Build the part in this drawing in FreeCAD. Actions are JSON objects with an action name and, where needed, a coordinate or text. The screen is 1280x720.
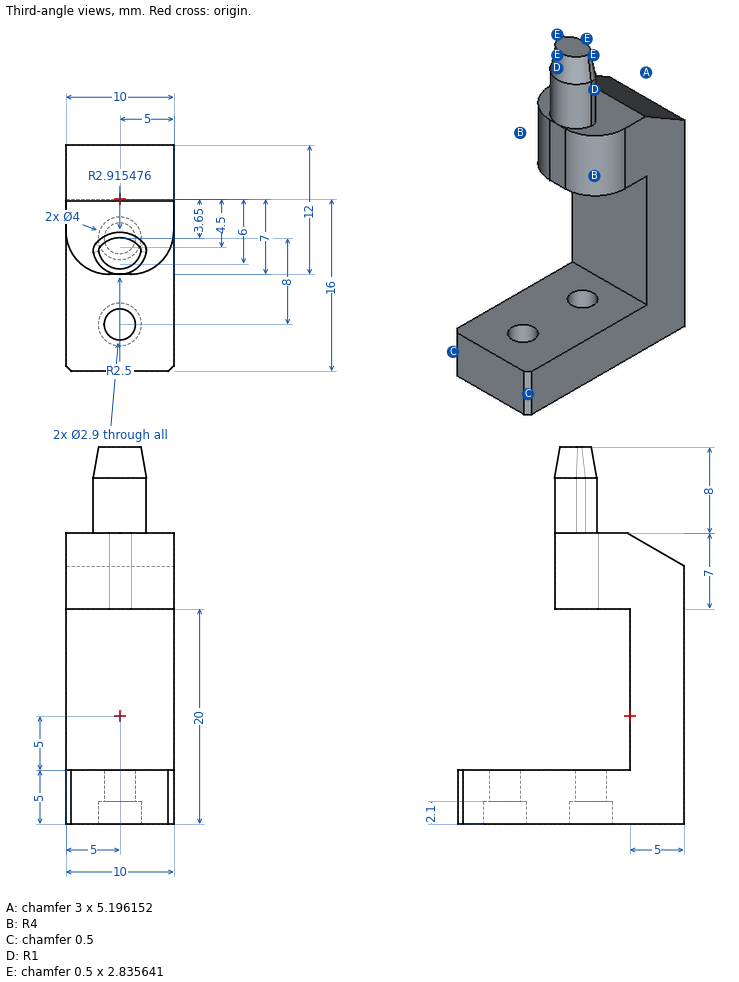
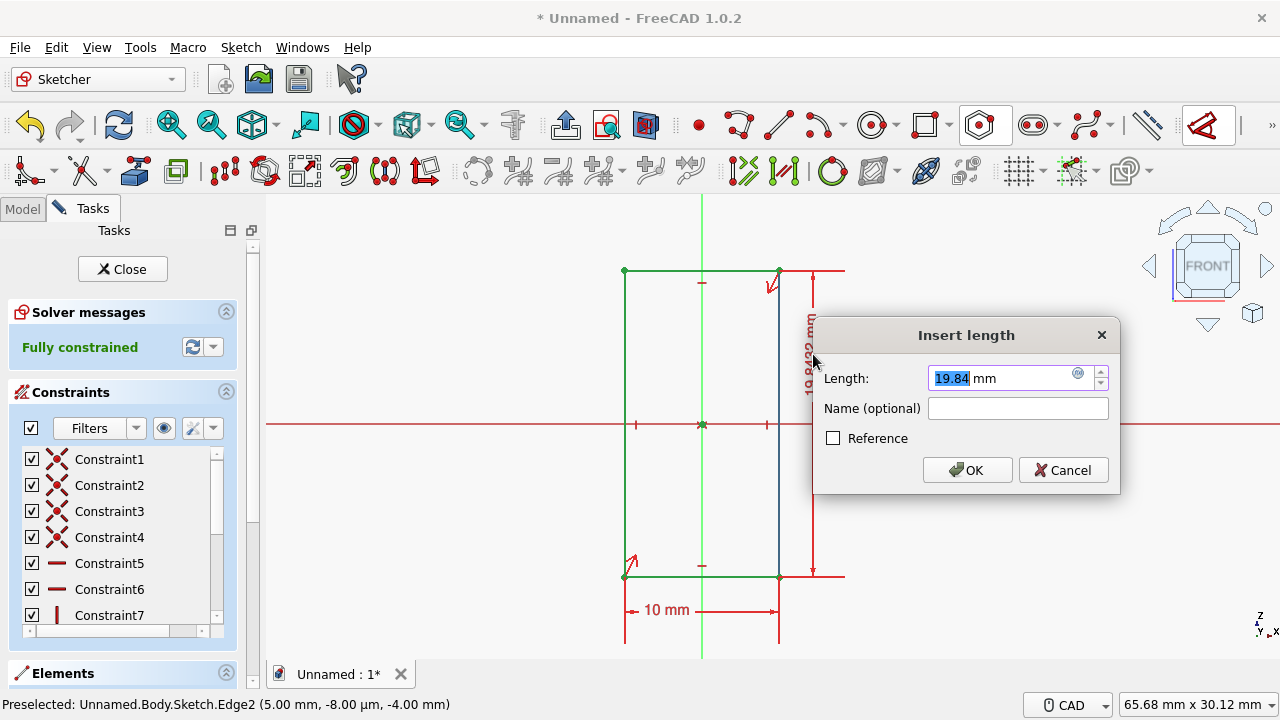
{"action": "type", "text": "20"}
{"action": "key", "text": "Return"}
{"action": "key", "text": "Escape"}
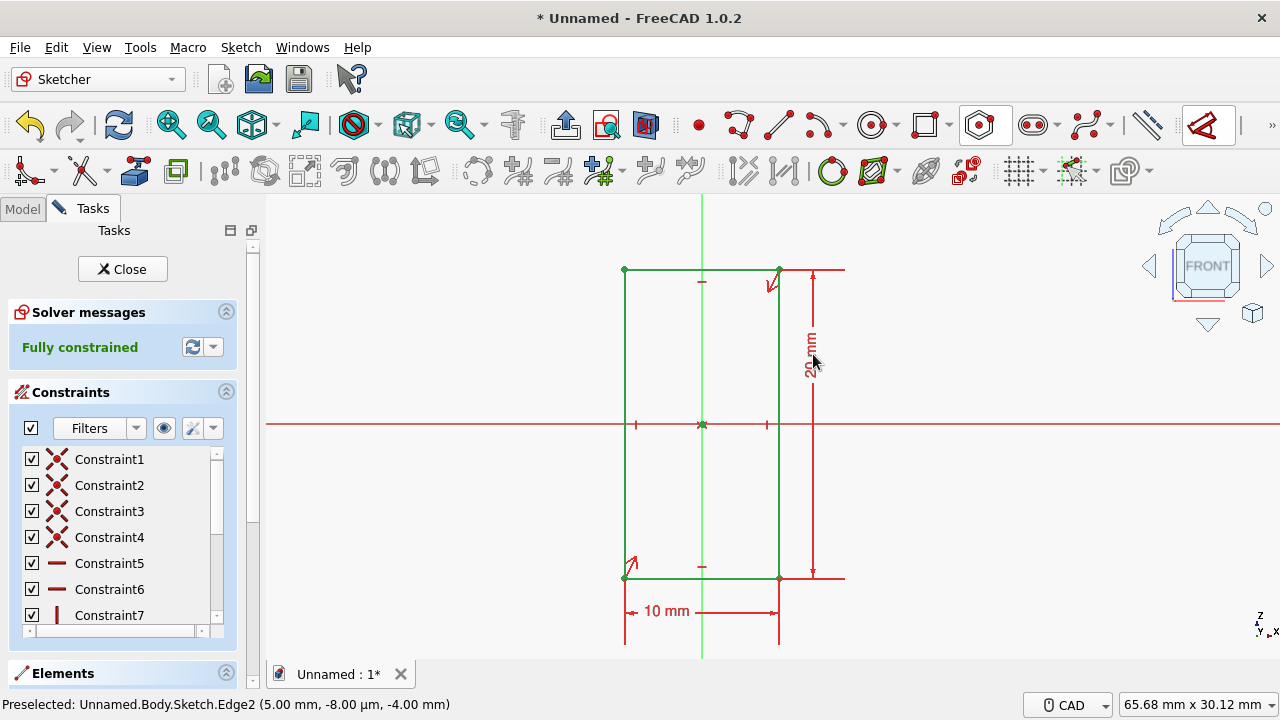
{"action": "left_click", "coordinate": [123, 269]}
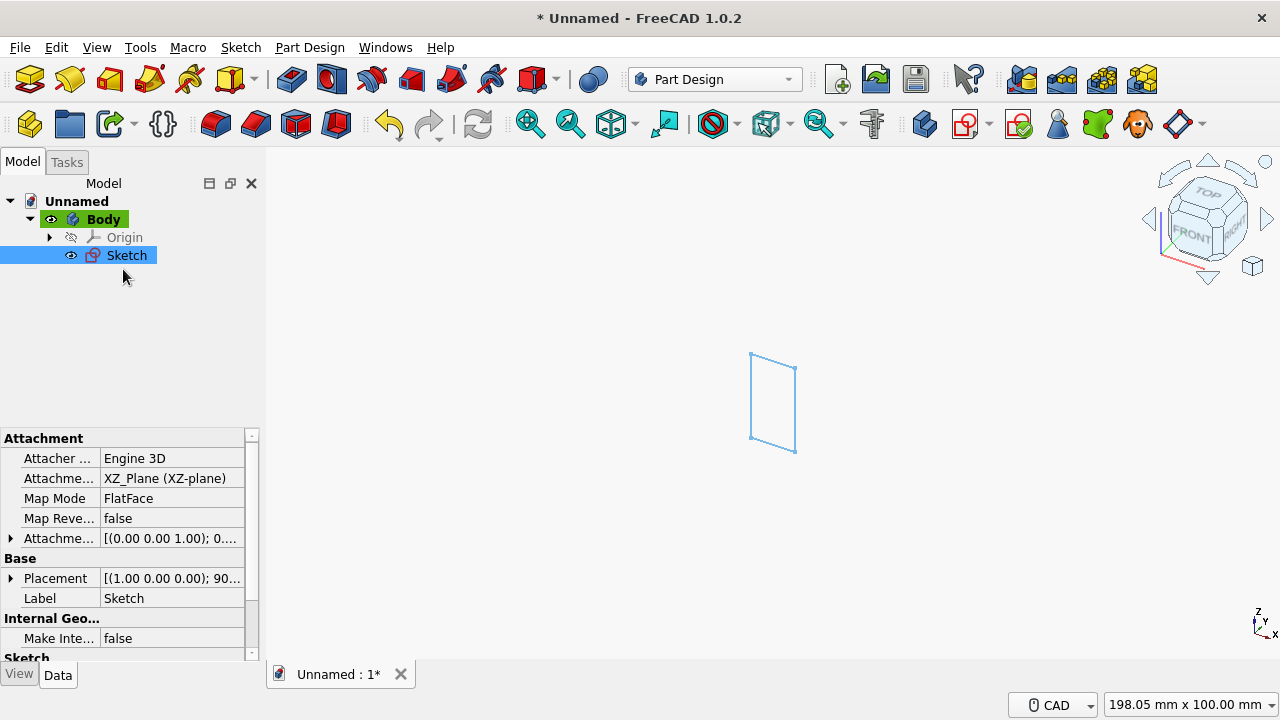
{"action": "left_click", "coordinate": [30, 80]}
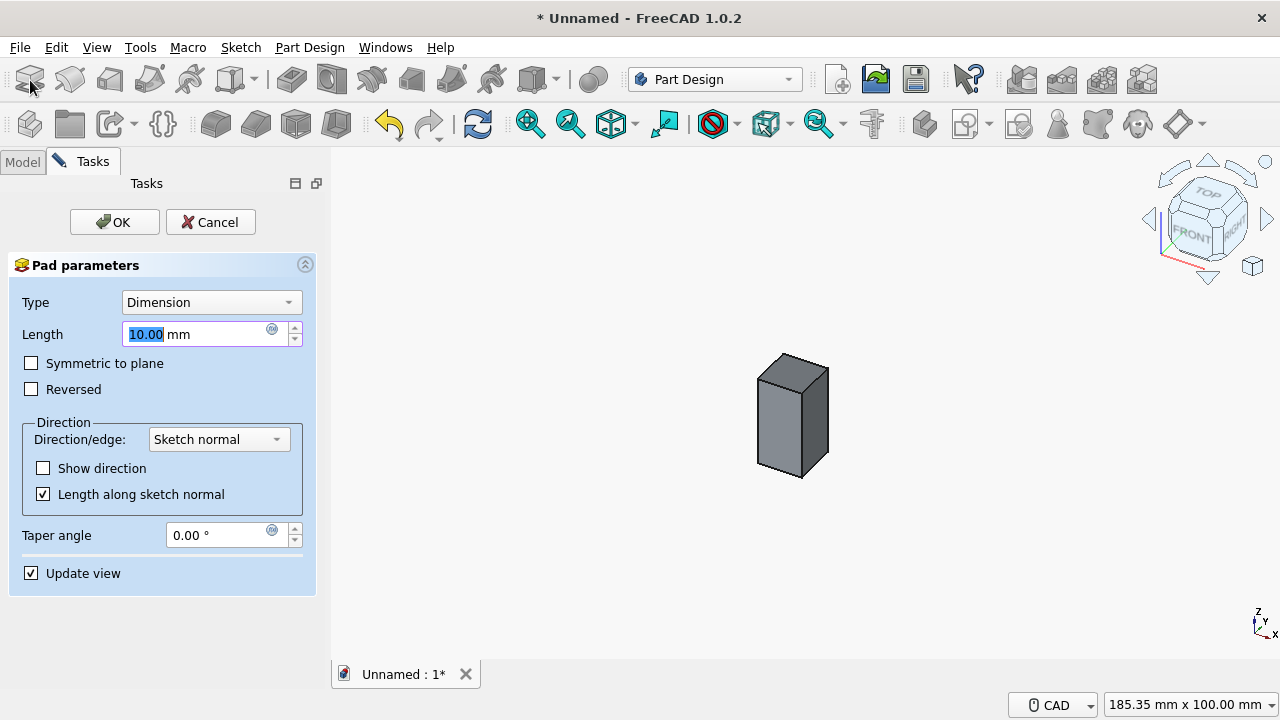
{"action": "type", "text": "5"}
{"action": "key", "text": "Tab"}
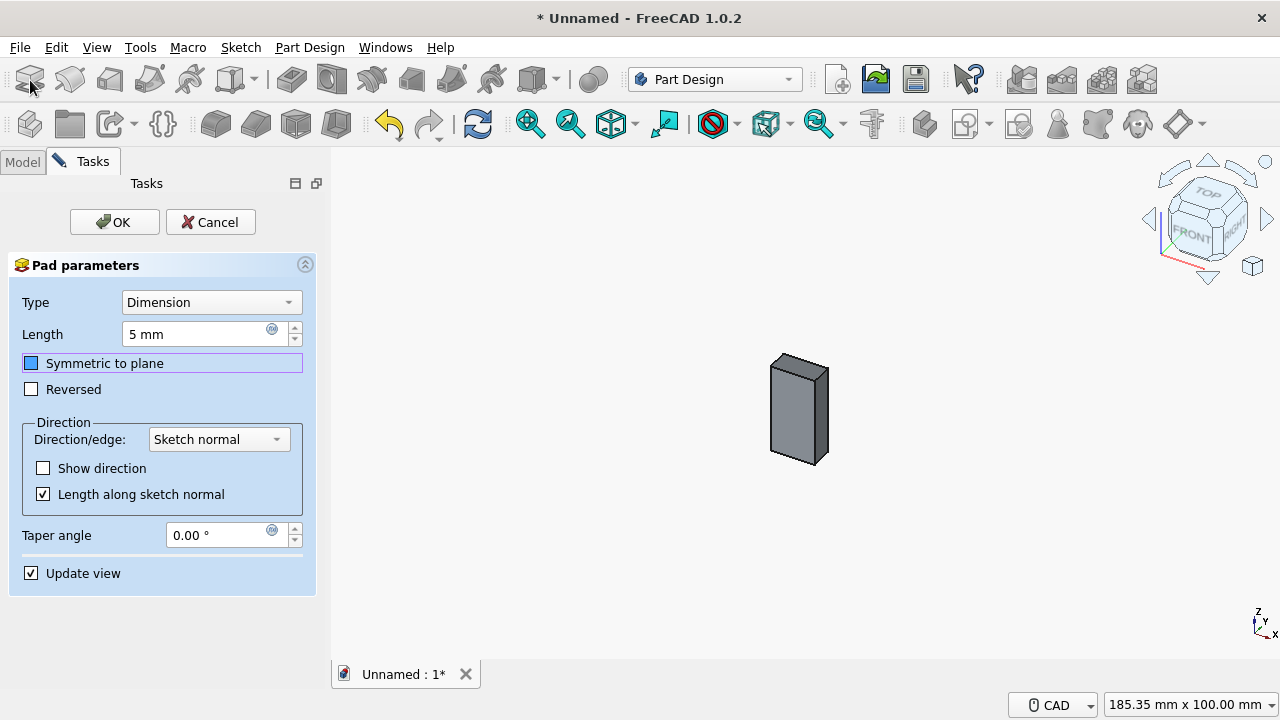
{"action": "left_click", "coordinate": [30, 389]}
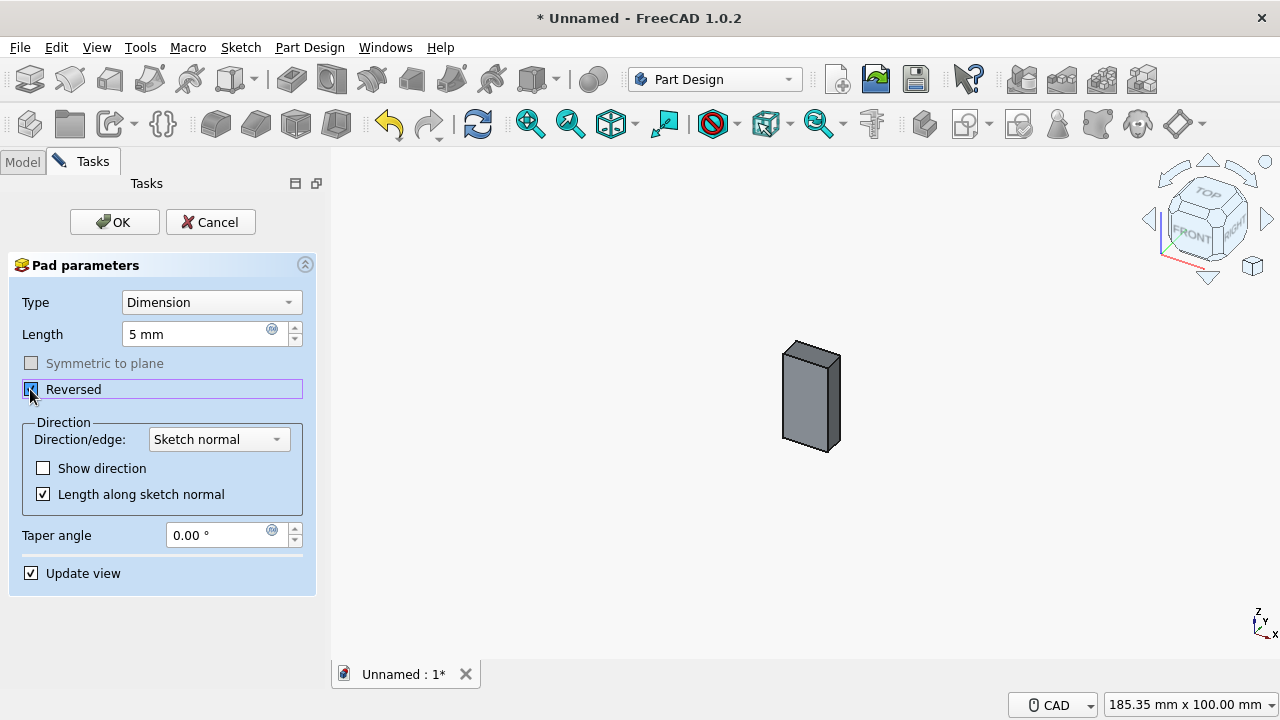
{"action": "left_click", "coordinate": [115, 222]}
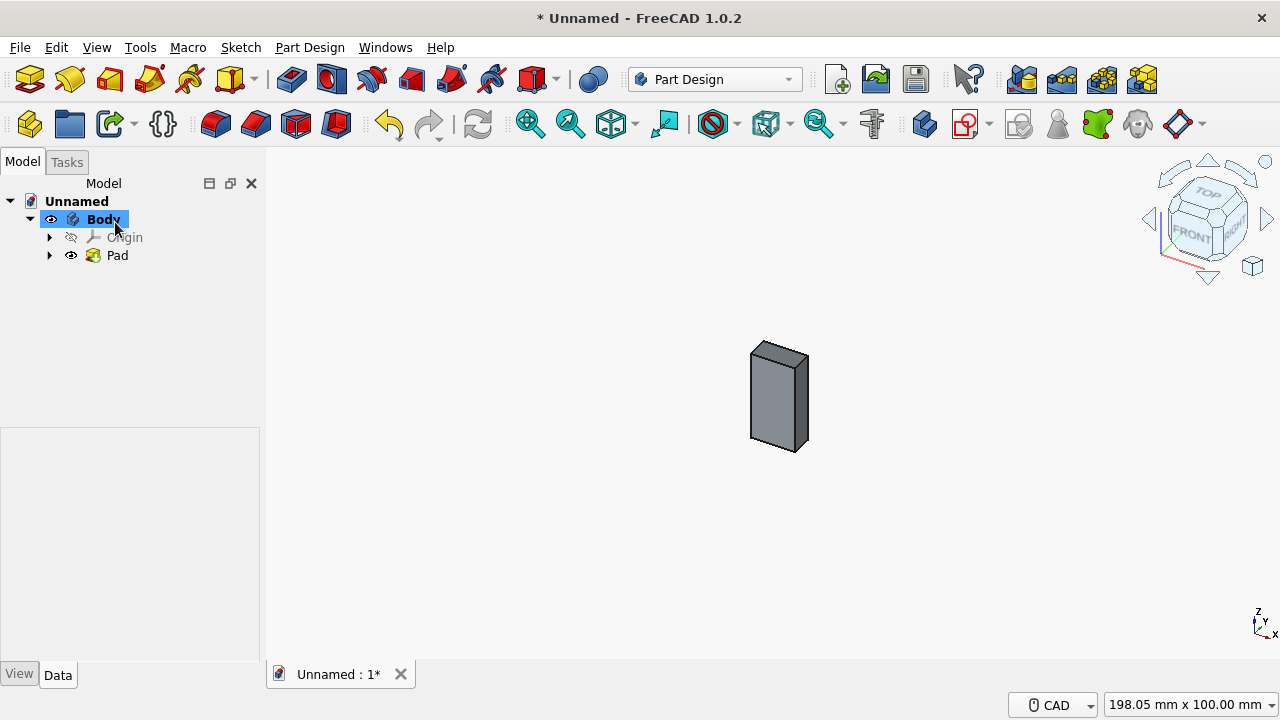
{"action": "left_click", "coordinate": [532, 124]}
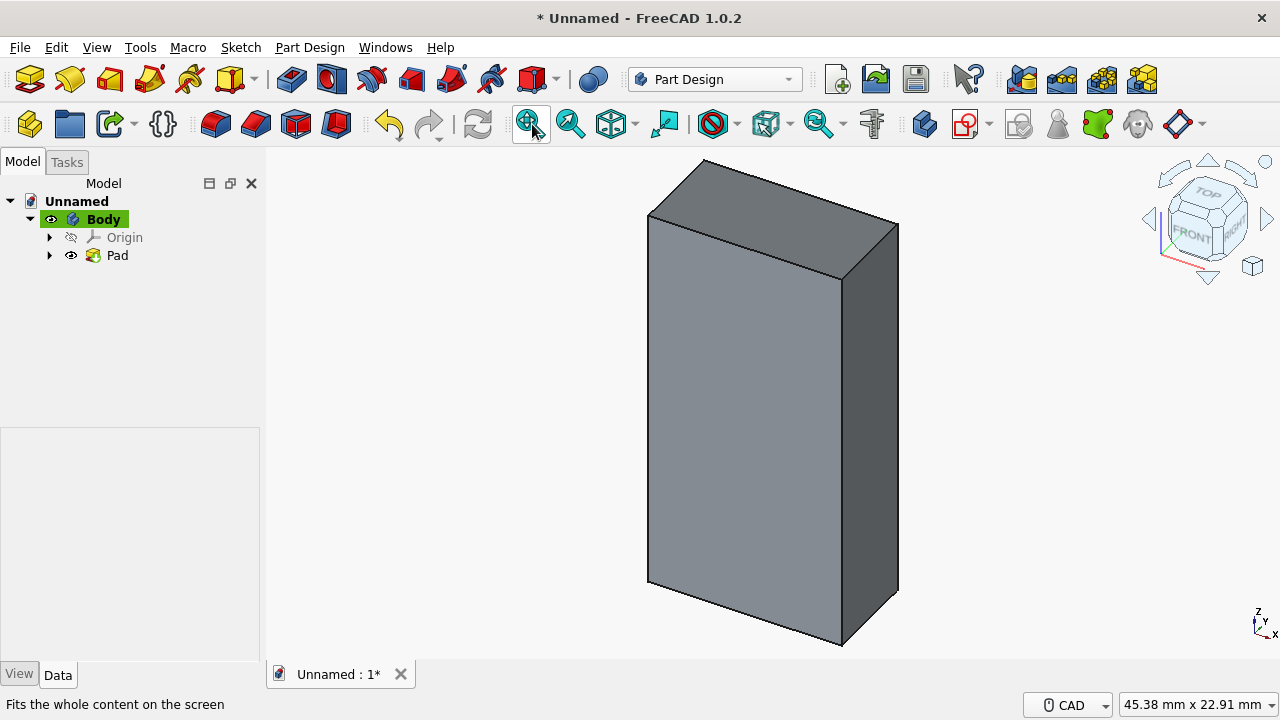
{"action": "left_click", "coordinate": [745, 377]}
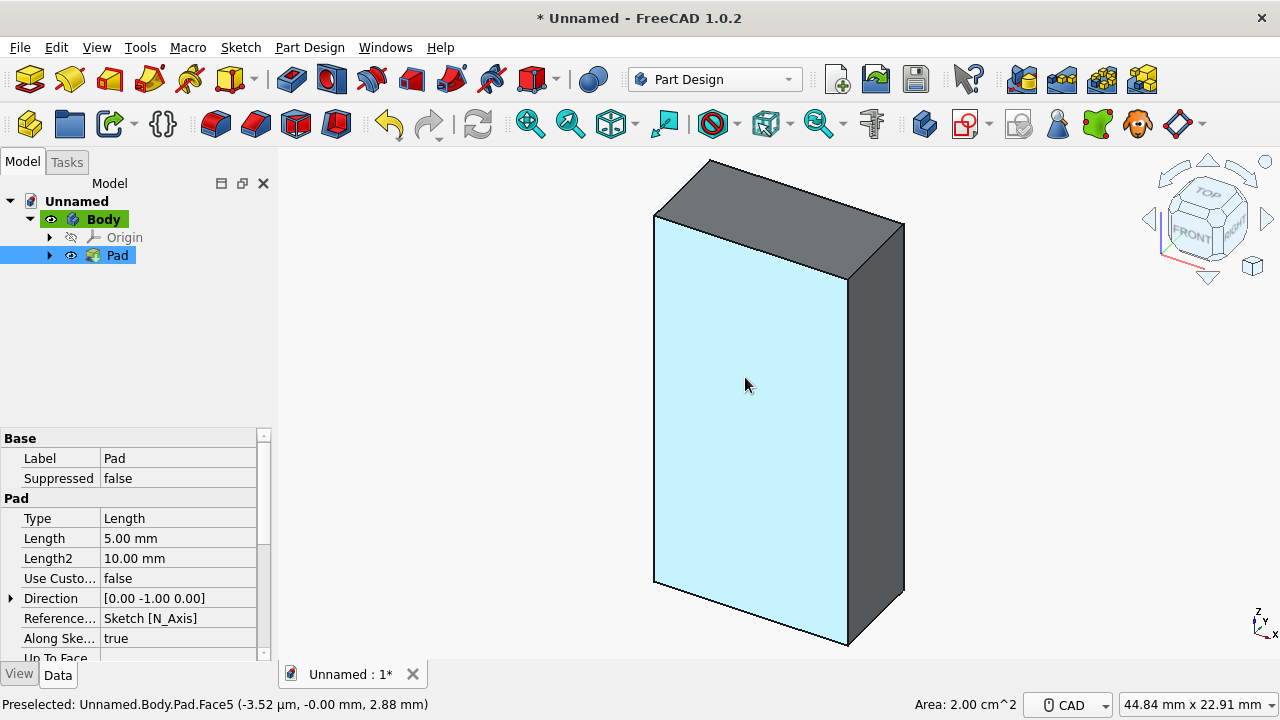
{"action": "left_click", "coordinate": [966, 124]}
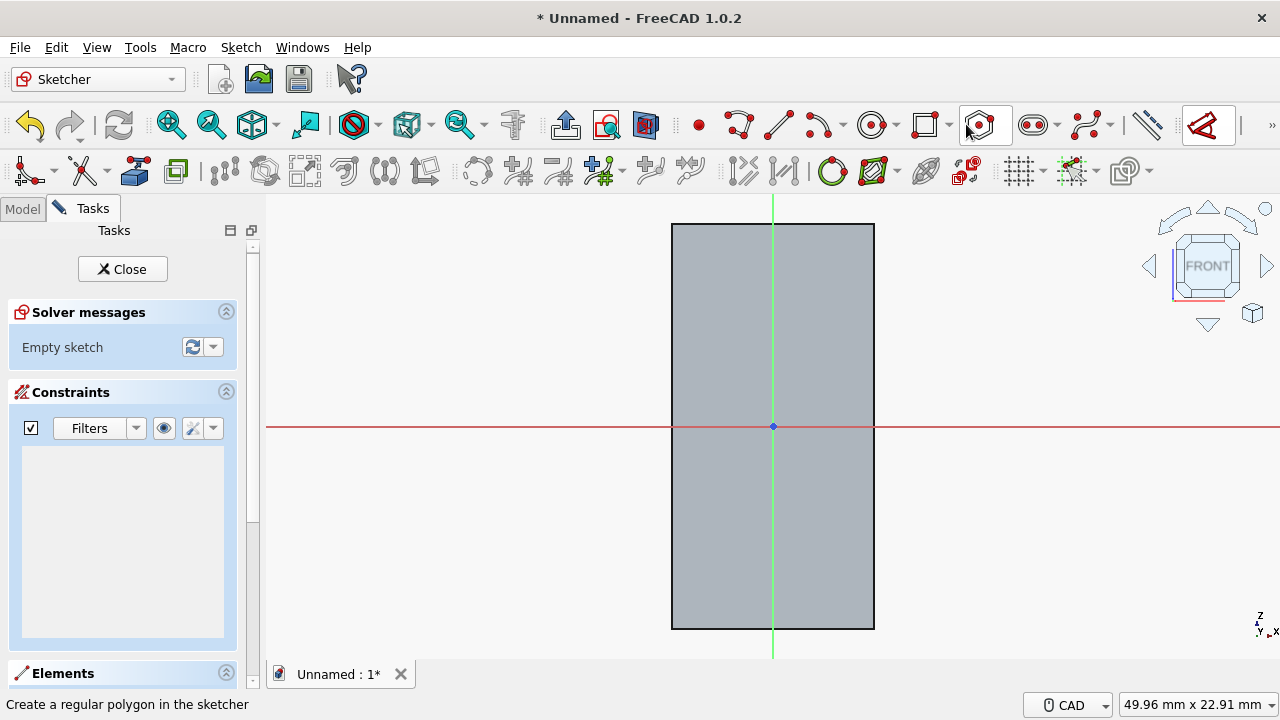
{"action": "scroll", "coordinate": [395, 222], "scroll_direction": "down", "scroll_amount": 1}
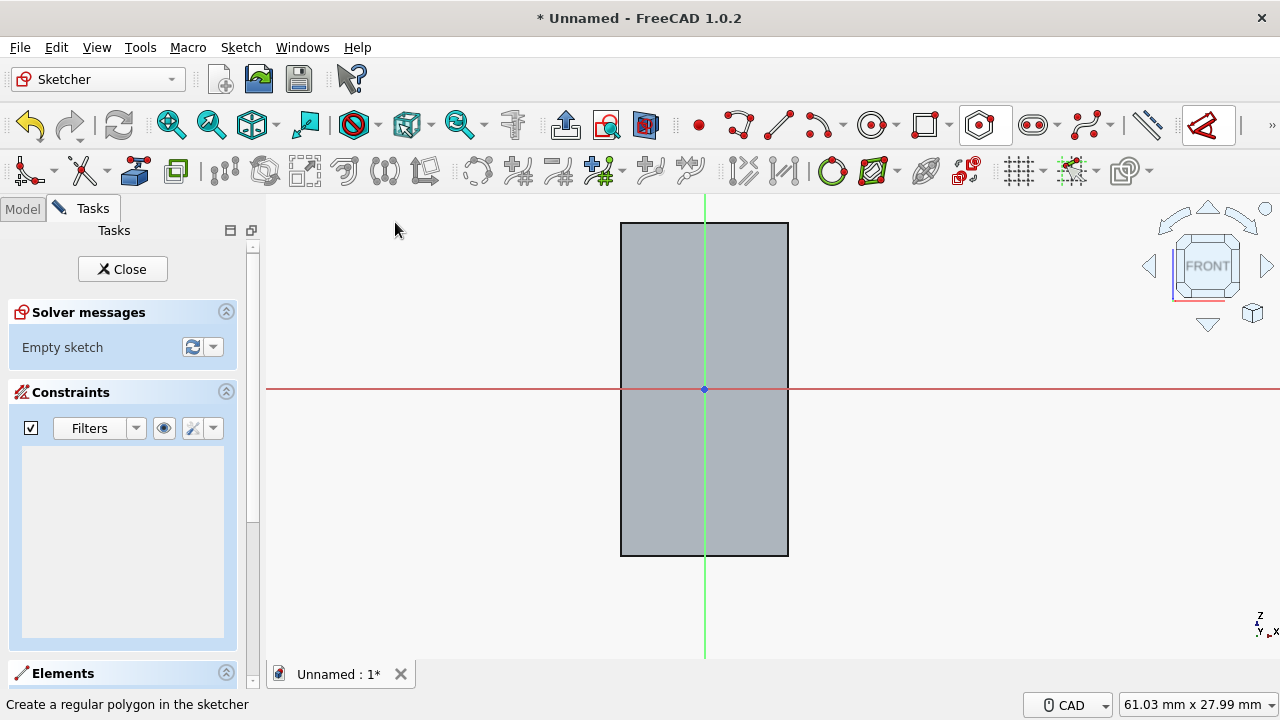
{"action": "scroll", "coordinate": [705, 528], "scroll_direction": "up", "scroll_amount": 3}